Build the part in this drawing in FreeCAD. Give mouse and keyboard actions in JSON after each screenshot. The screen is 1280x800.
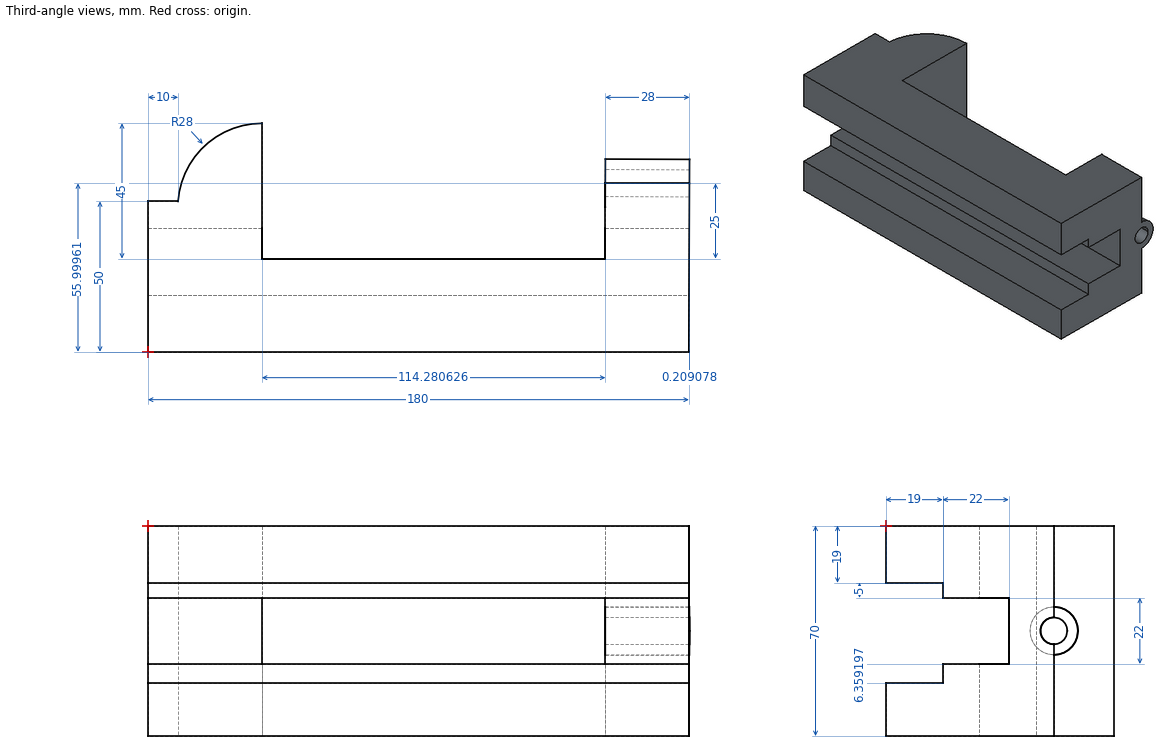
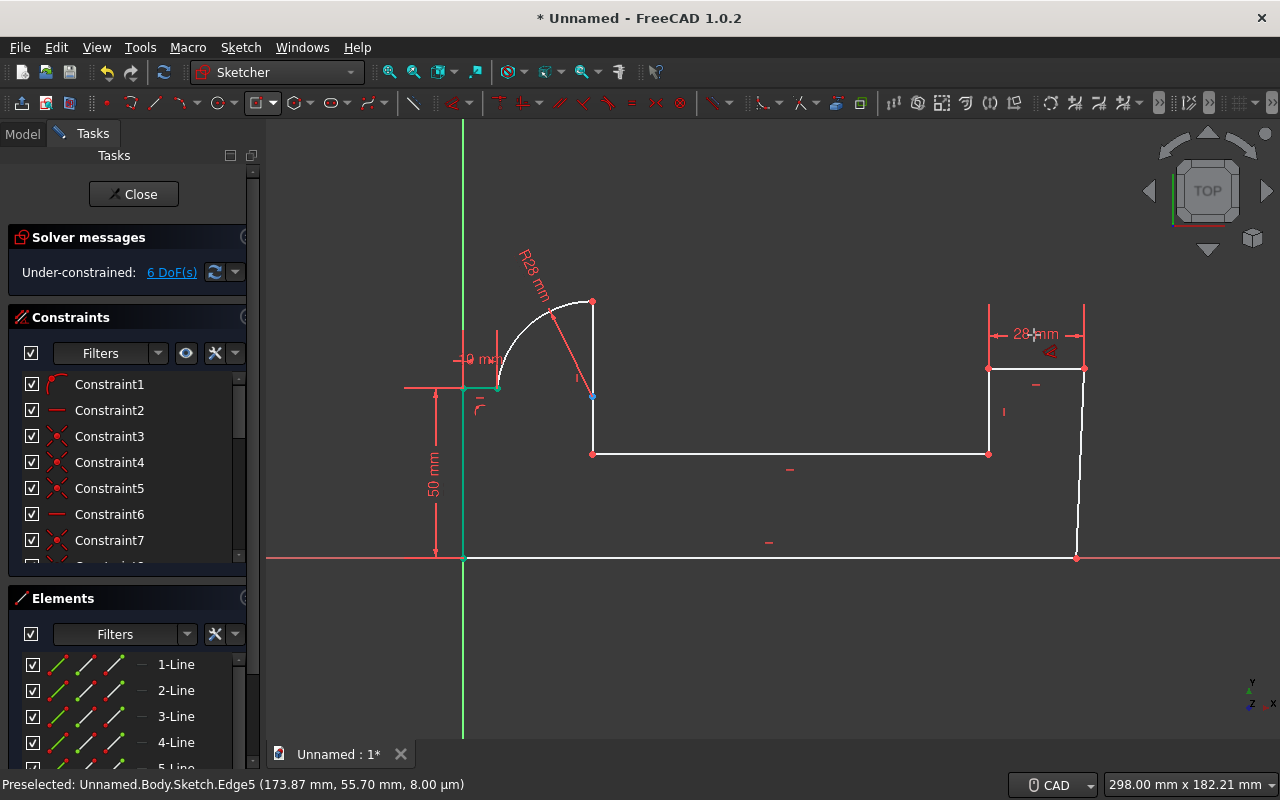
{"action": "left_click", "coordinate": [989, 395]}
{"action": "left_click", "coordinate": [1023, 412]}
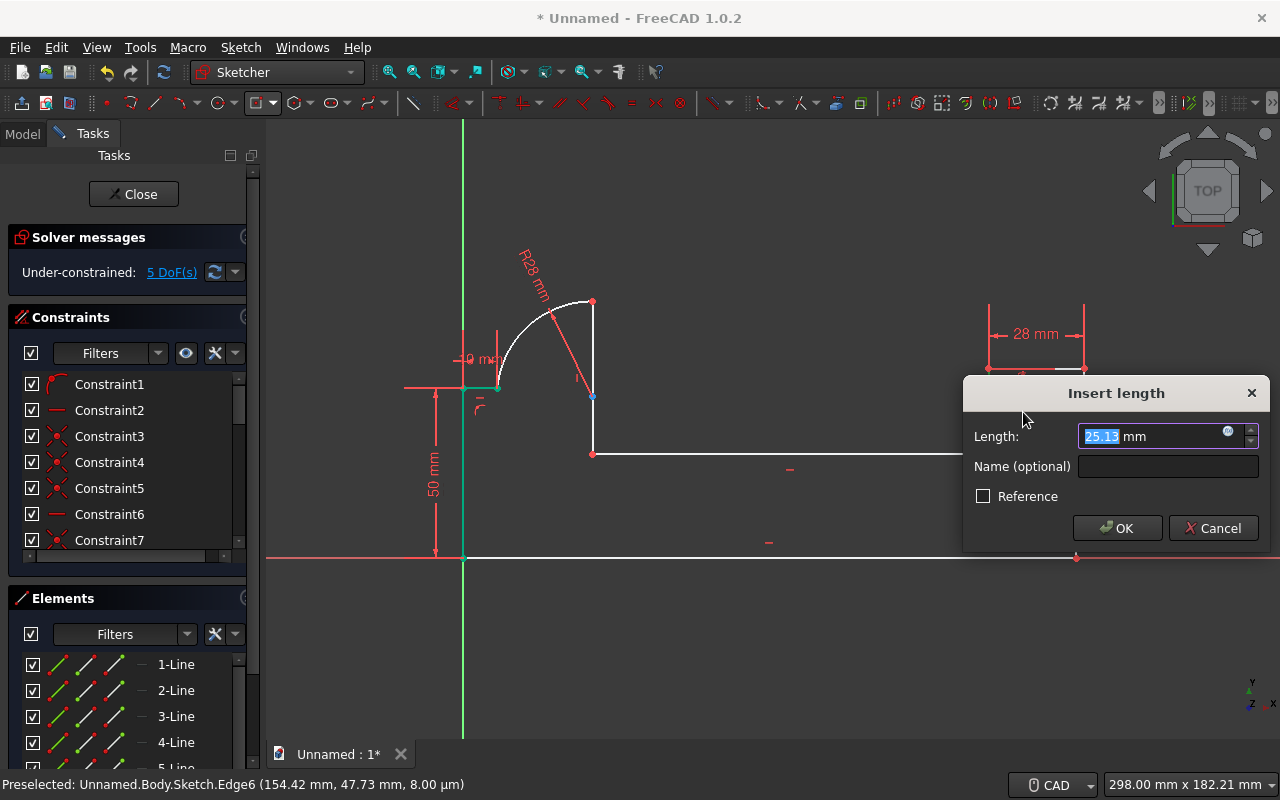
{"action": "type", "text": "25"}
{"action": "key", "text": "Return"}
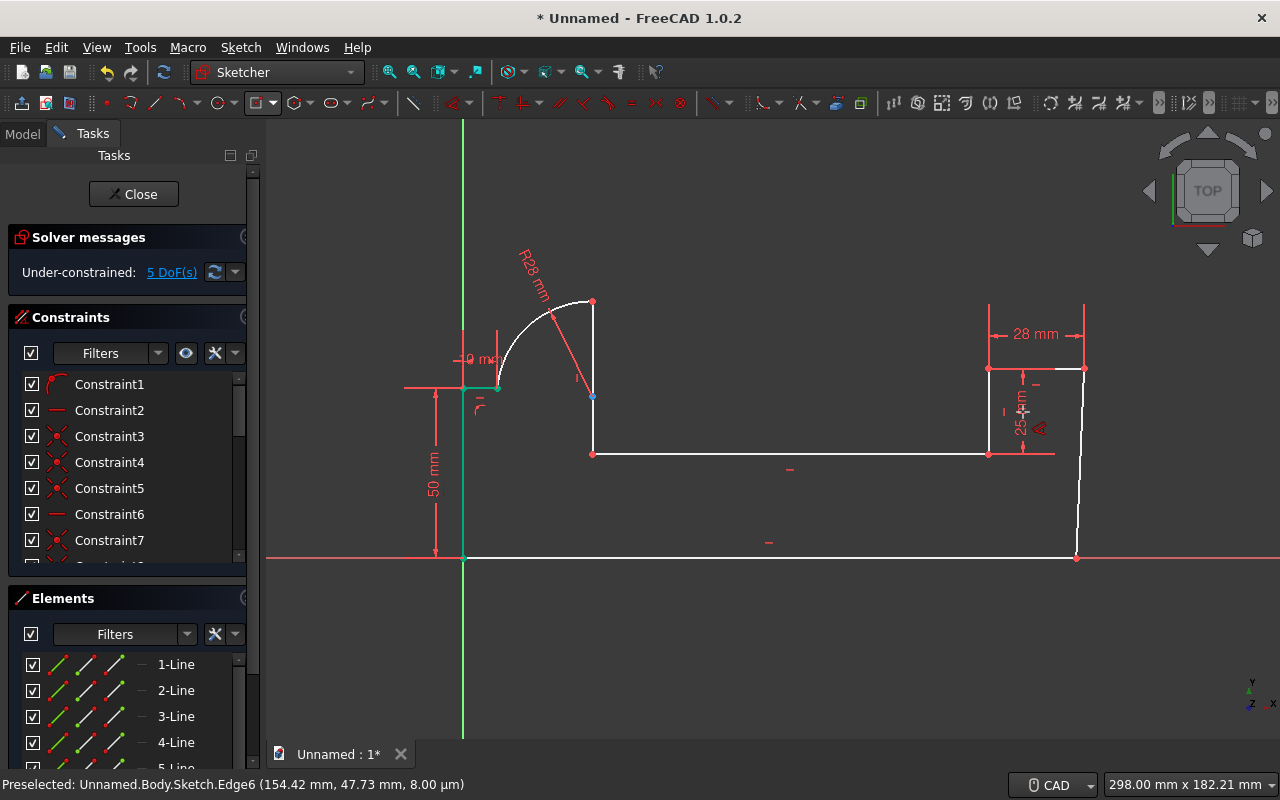
{"action": "left_click", "coordinate": [593, 408]}
{"action": "left_click", "coordinate": [559, 378]}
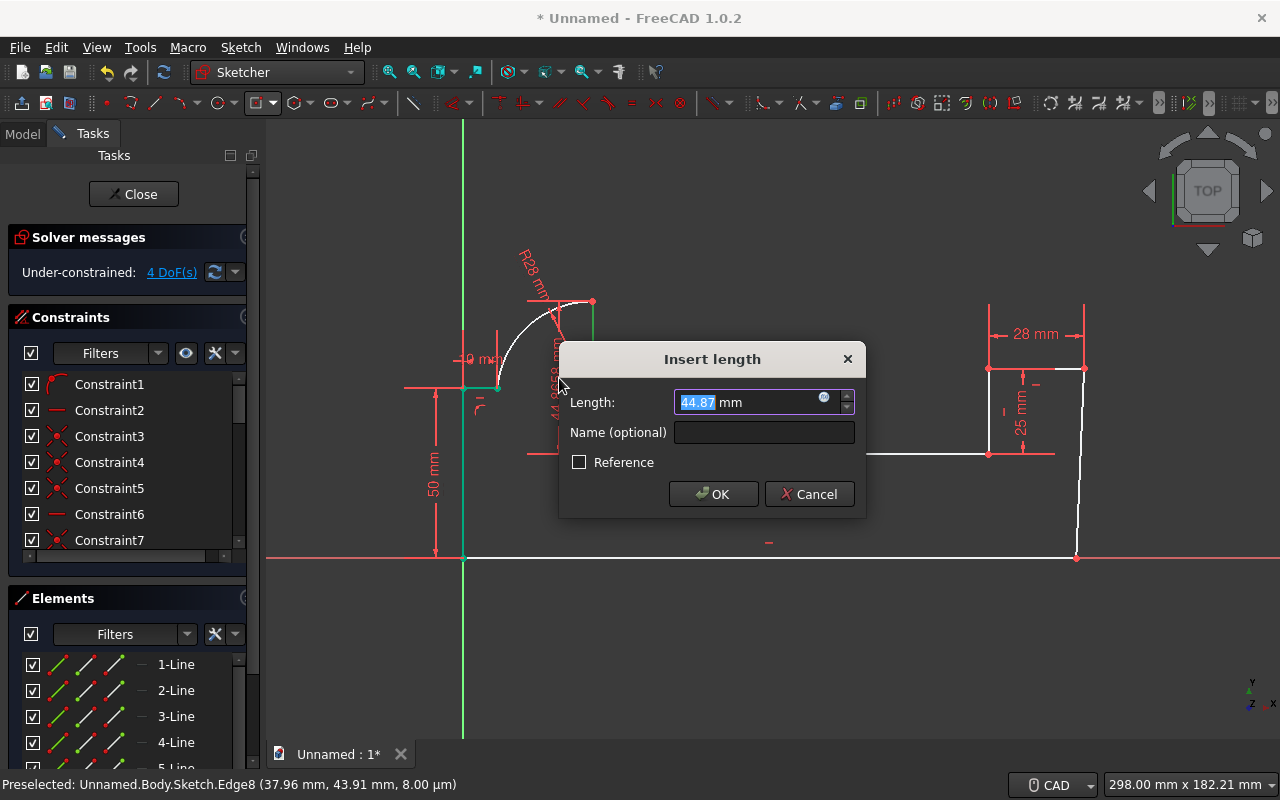
{"action": "type", "text": "45"}
{"action": "key", "text": "Return"}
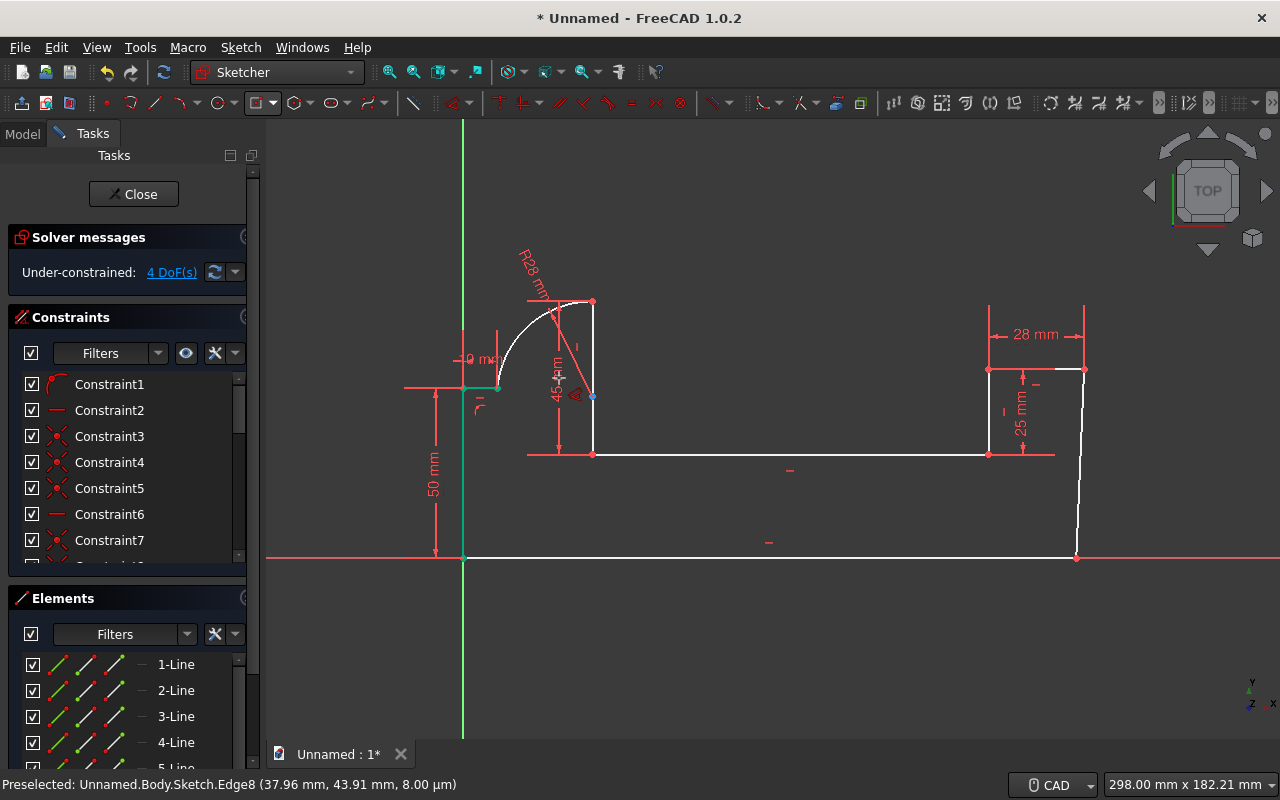
{"action": "left_click", "coordinate": [647, 558]}
{"action": "left_click", "coordinate": [770, 592]}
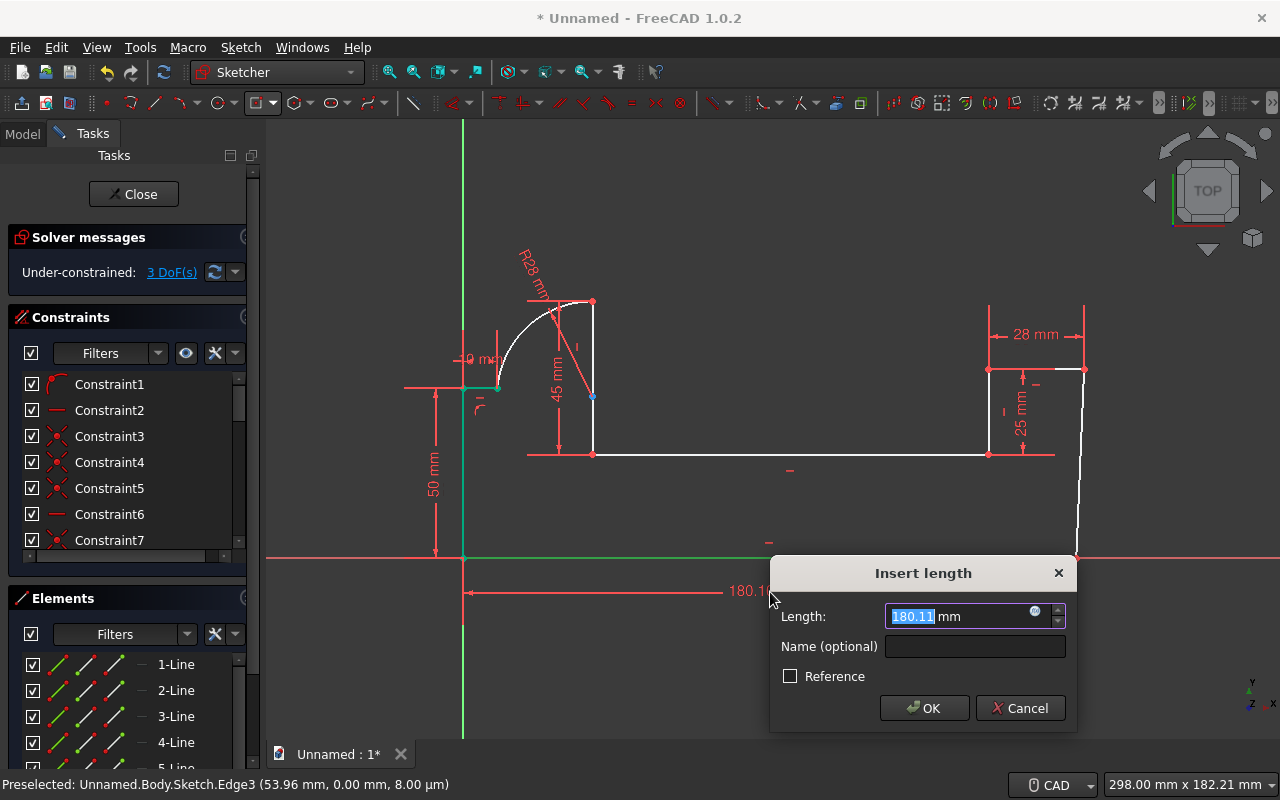
{"action": "type", "text": "180"}
{"action": "key", "text": "Return"}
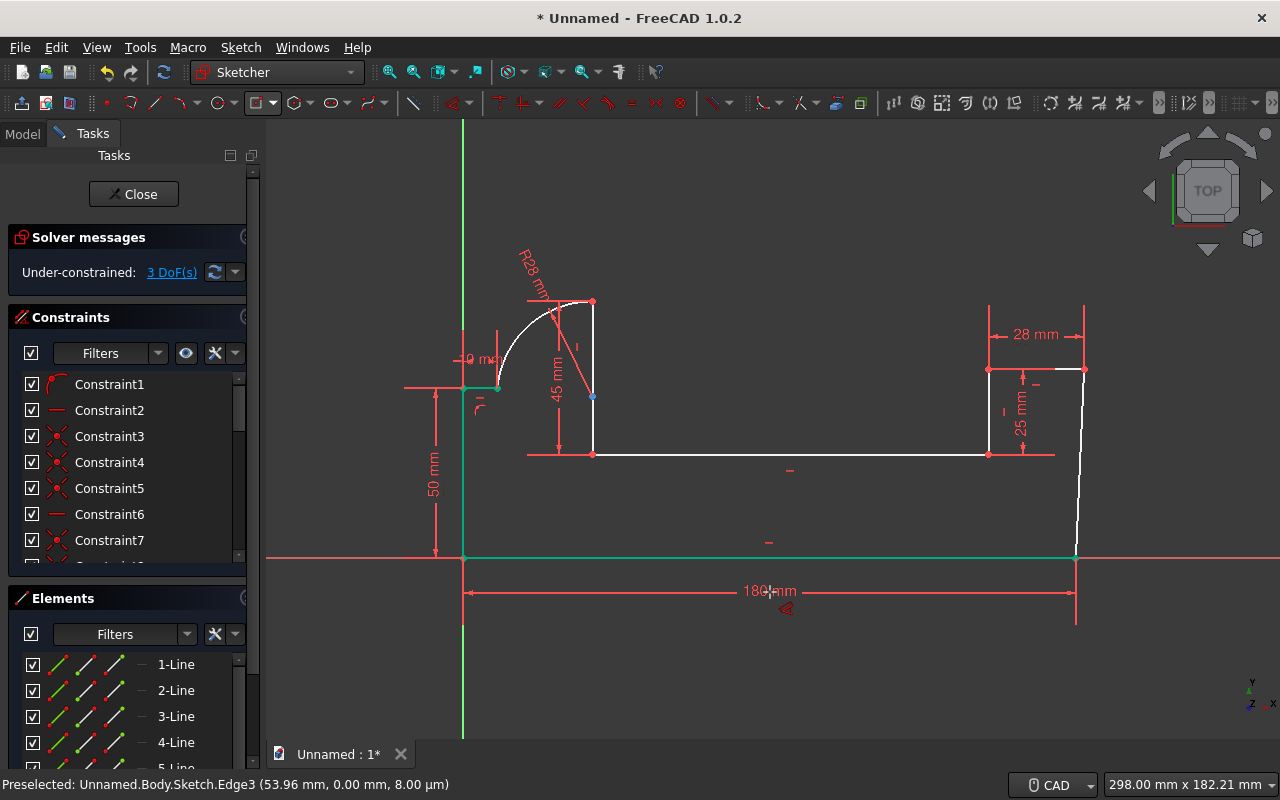
{"action": "left_click", "coordinate": [1084, 369]}
{"action": "left_click", "coordinate": [429, 420]}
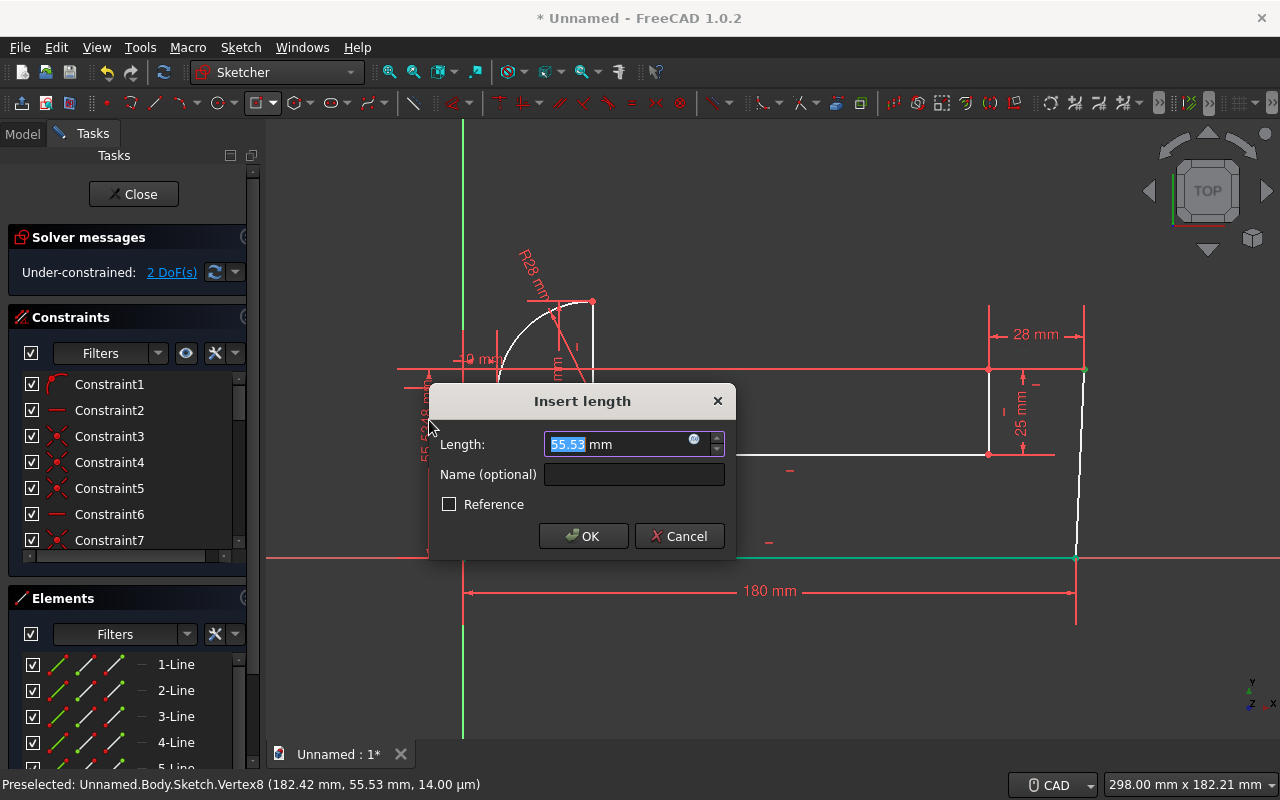
{"action": "type", "text": "55.99961"}
{"action": "key", "text": "Return"}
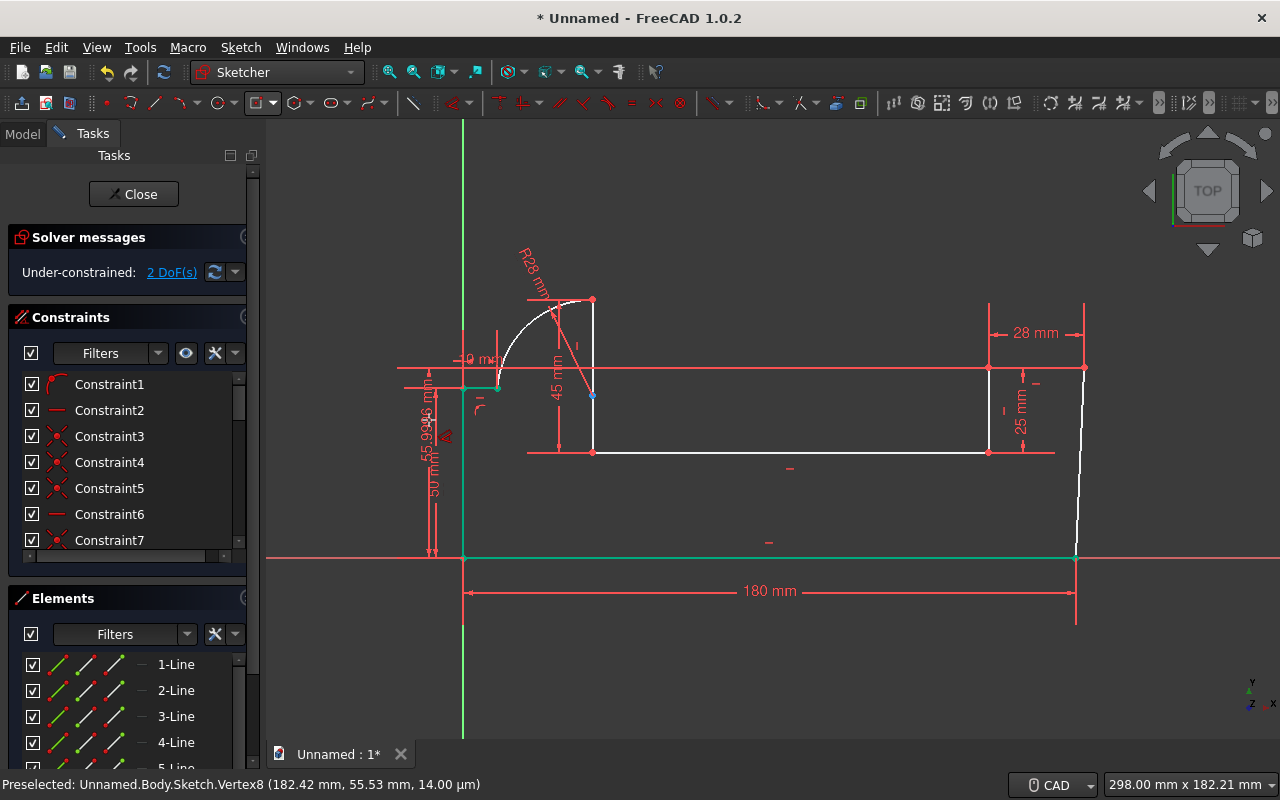
{"action": "scroll", "coordinate": [1078, 501], "scroll_direction": "up", "scroll_amount": 21}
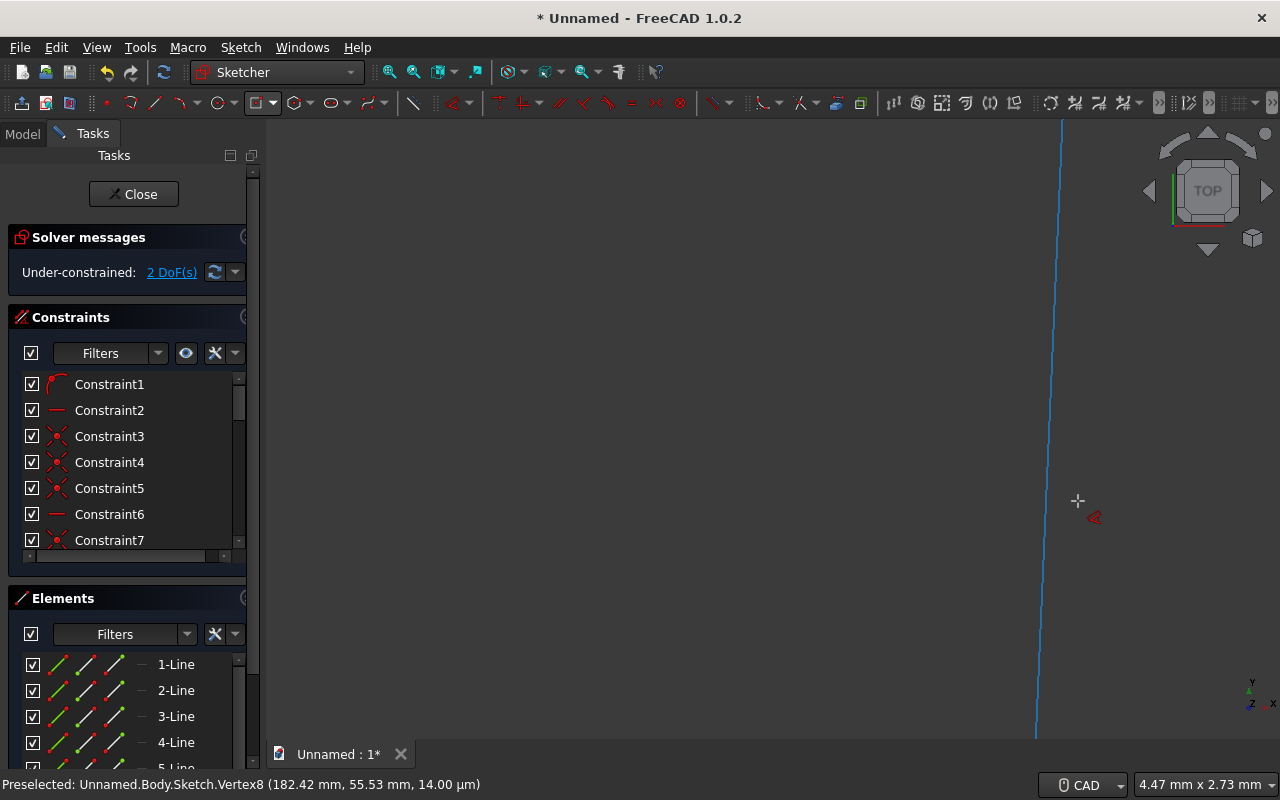
{"action": "left_click", "coordinate": [1047, 477]}